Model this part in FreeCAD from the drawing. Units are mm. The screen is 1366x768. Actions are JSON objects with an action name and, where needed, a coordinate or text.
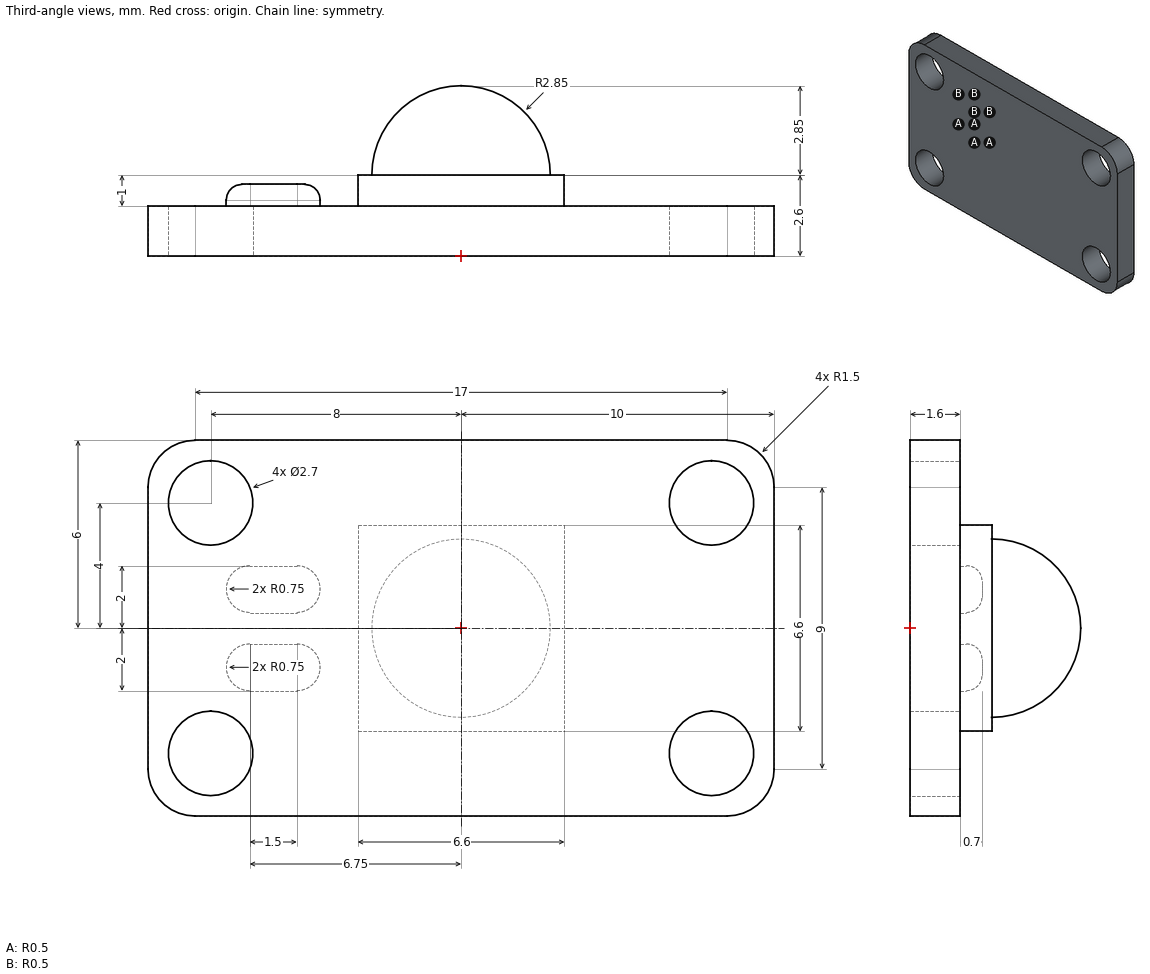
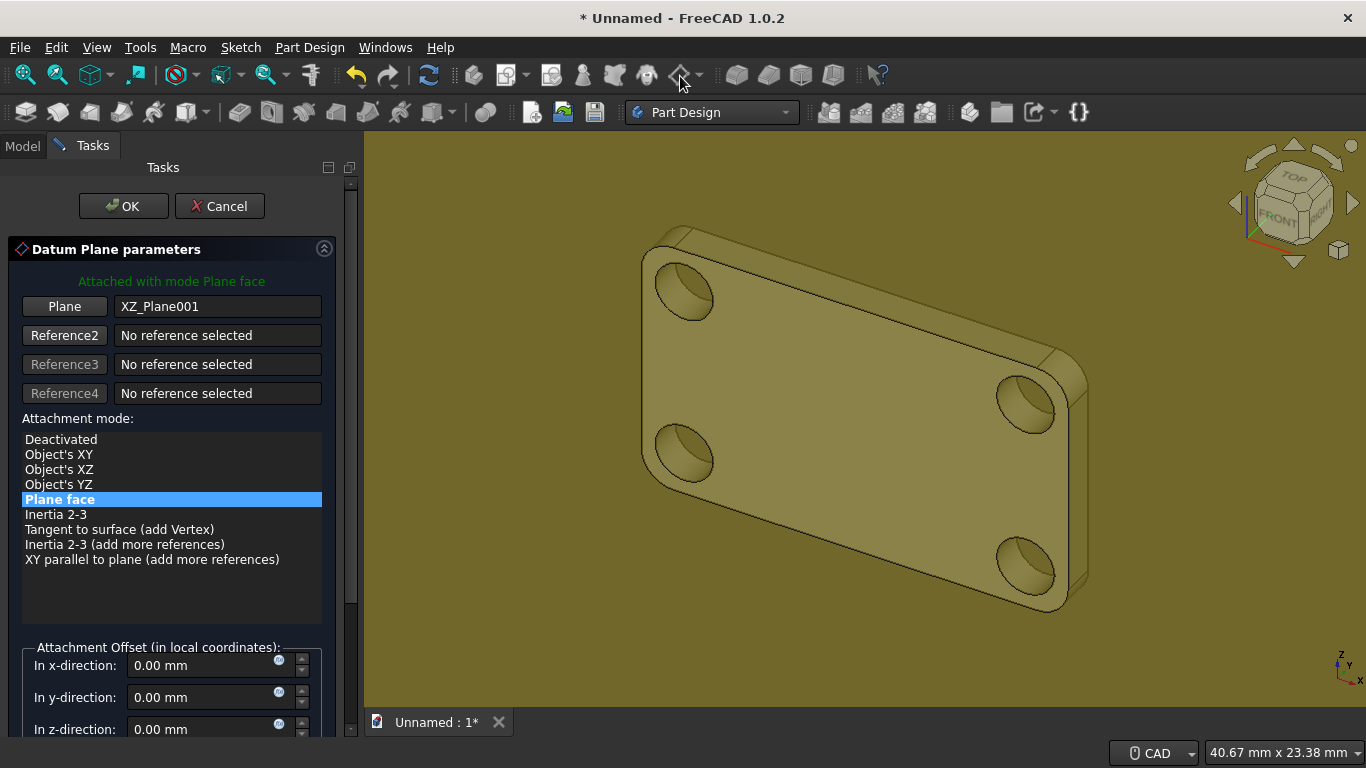
{"action": "scroll", "coordinate": [351, 456], "scroll_direction": "down", "scroll_amount": 2}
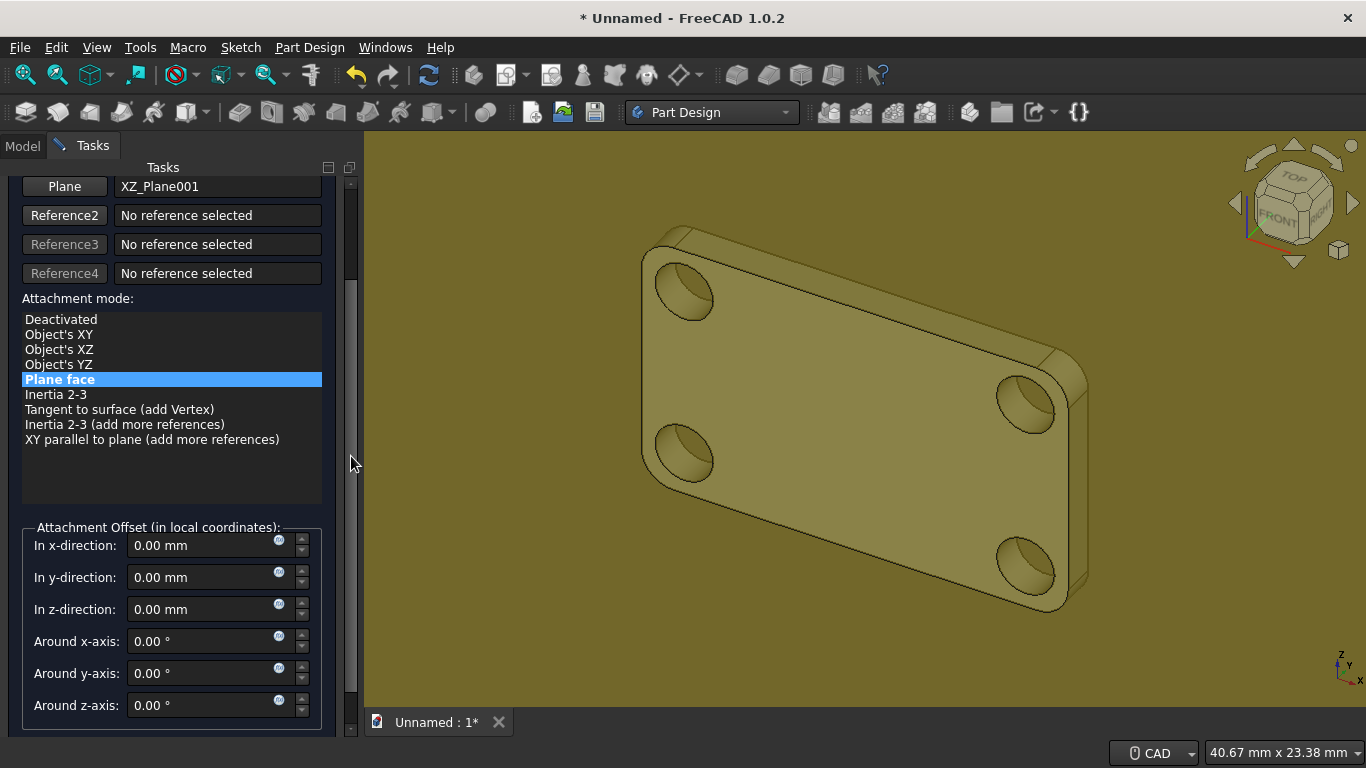
{"action": "triple_click", "coordinate": [210, 609]}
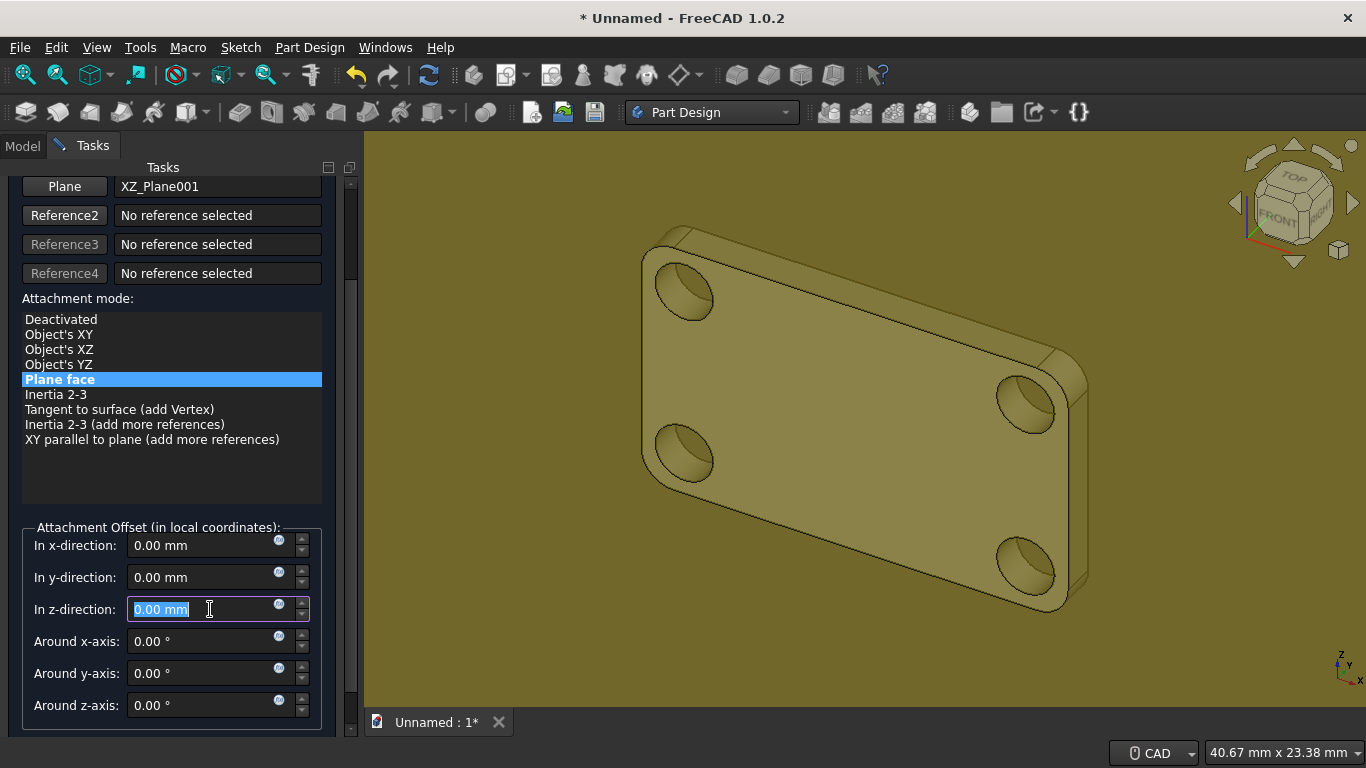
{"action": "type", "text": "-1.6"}
{"action": "key", "text": "Tab"}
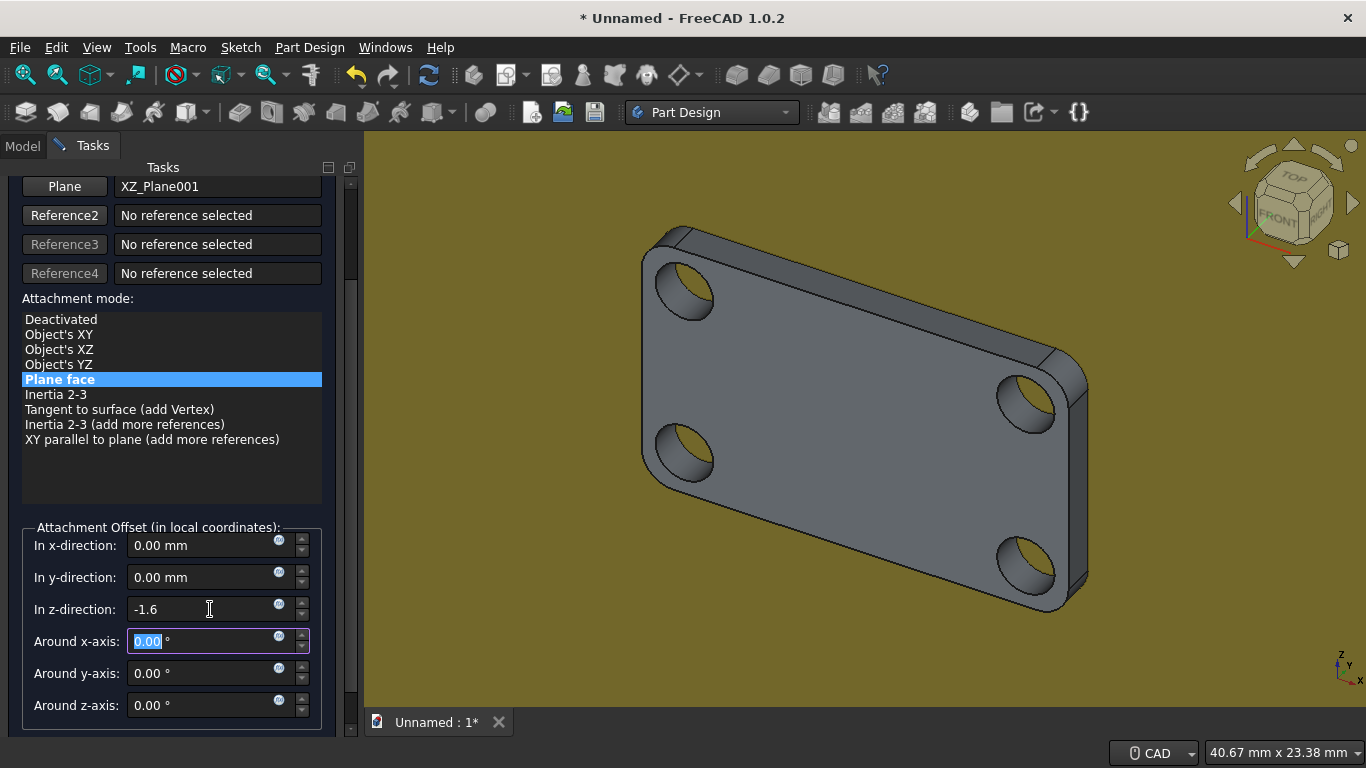
{"action": "scroll", "coordinate": [351, 456], "scroll_direction": "up", "scroll_amount": 3}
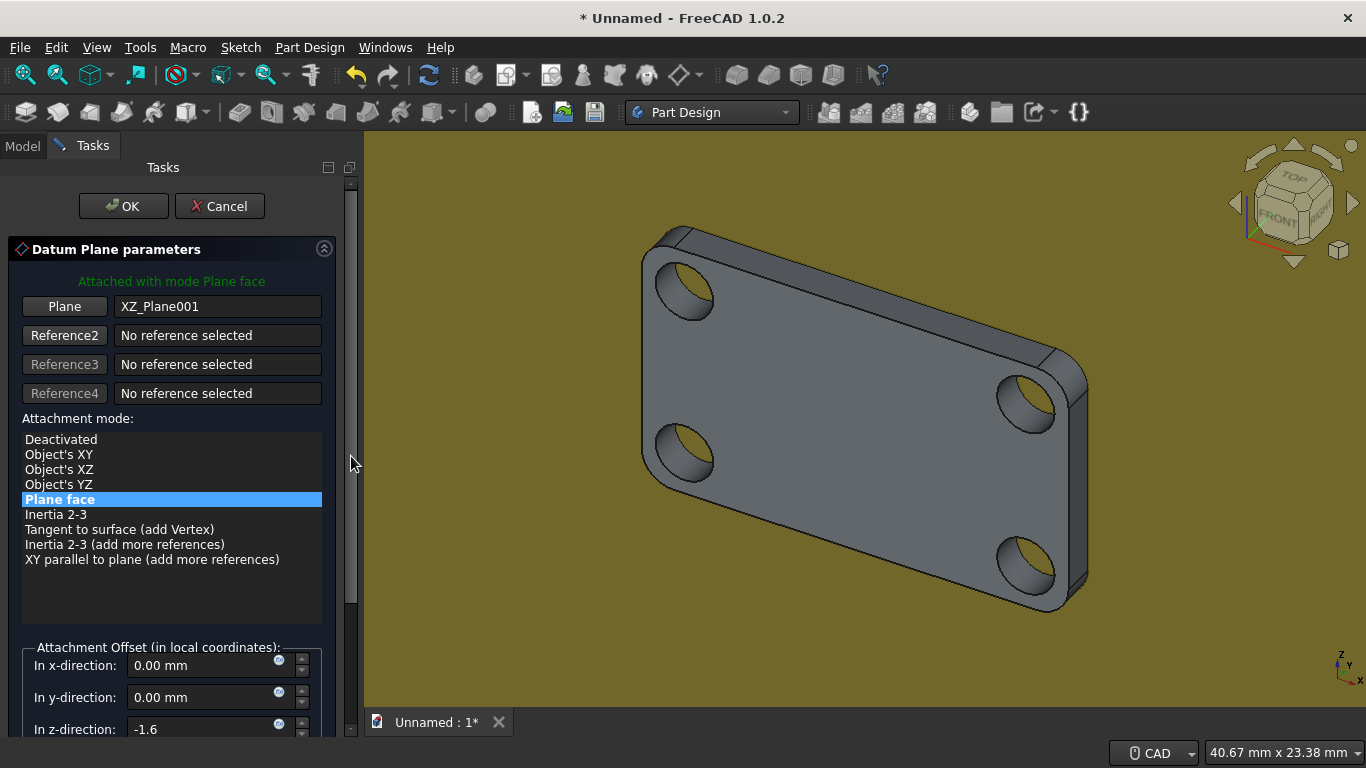
{"action": "left_click", "coordinate": [124, 206]}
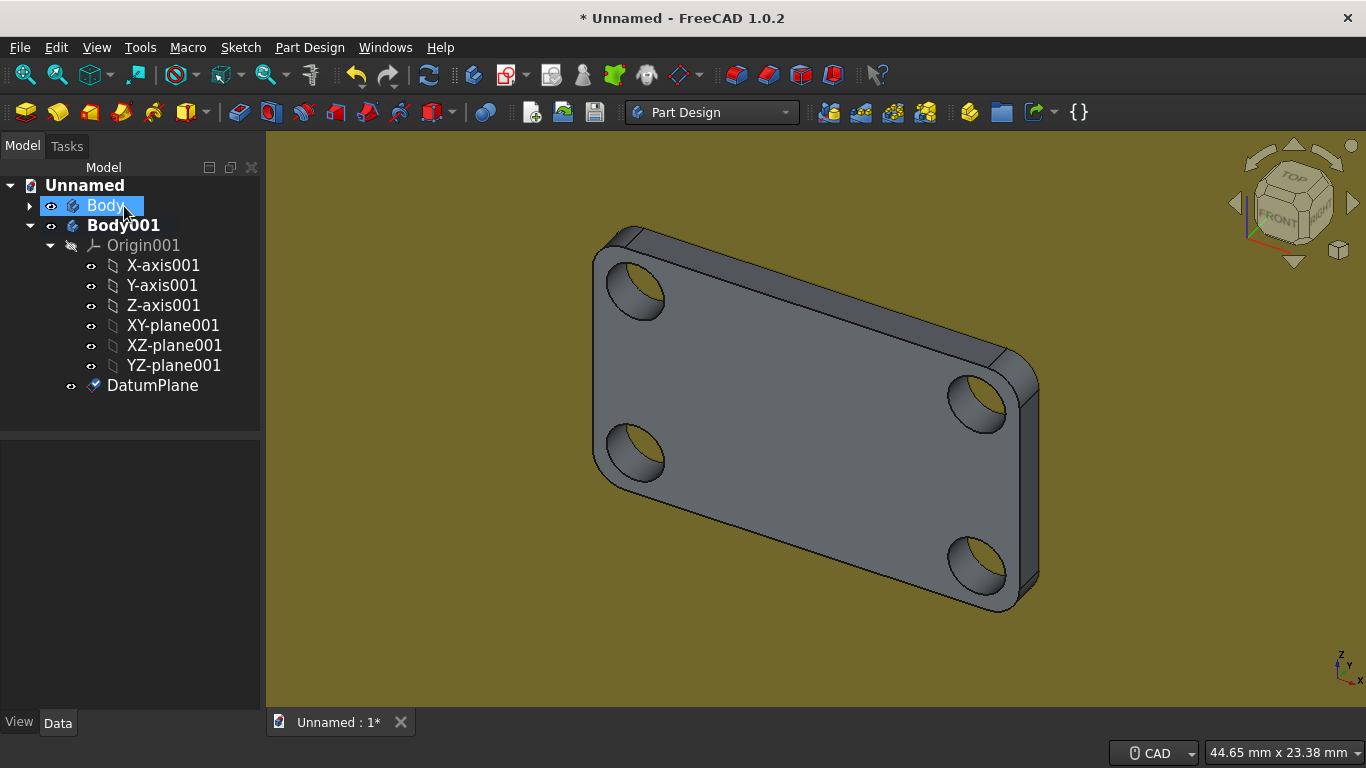
{"action": "left_click", "coordinate": [116, 386]}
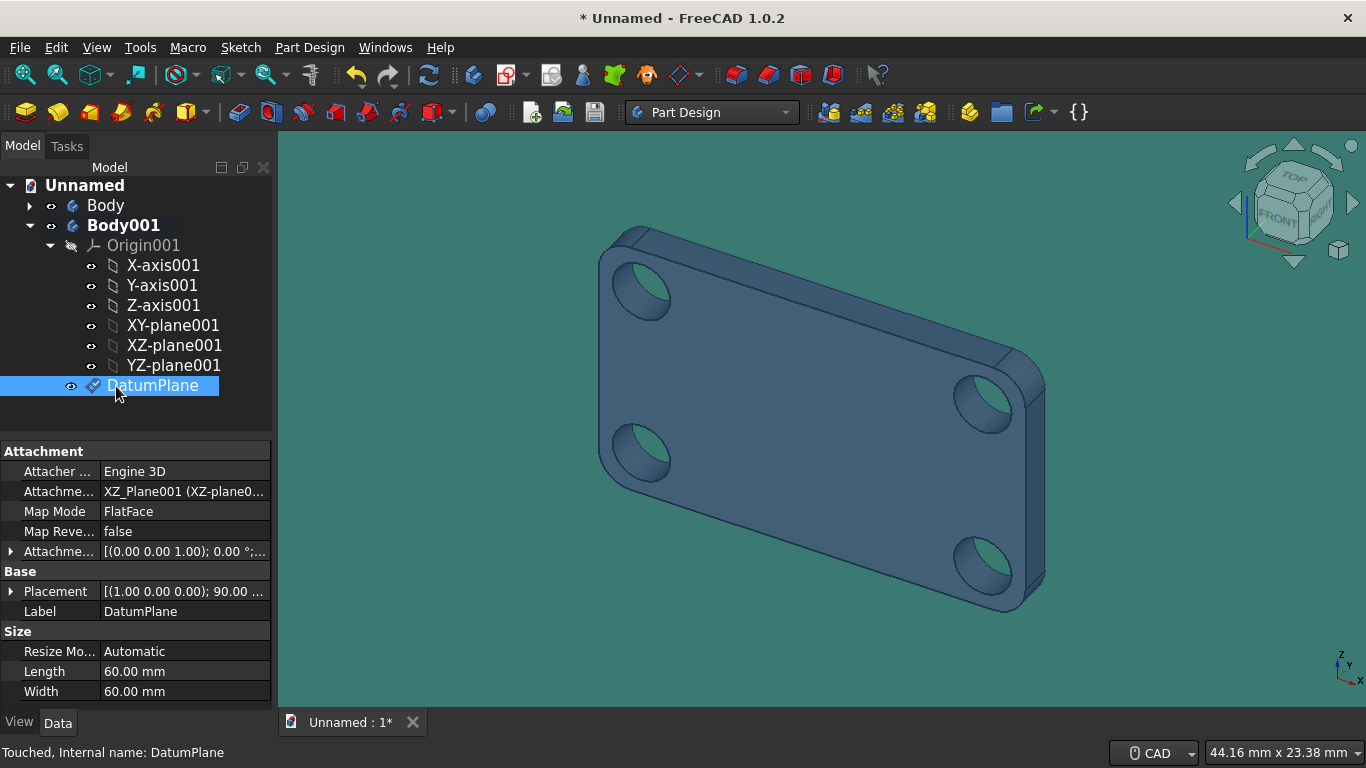
{"action": "left_click", "coordinate": [506, 76]}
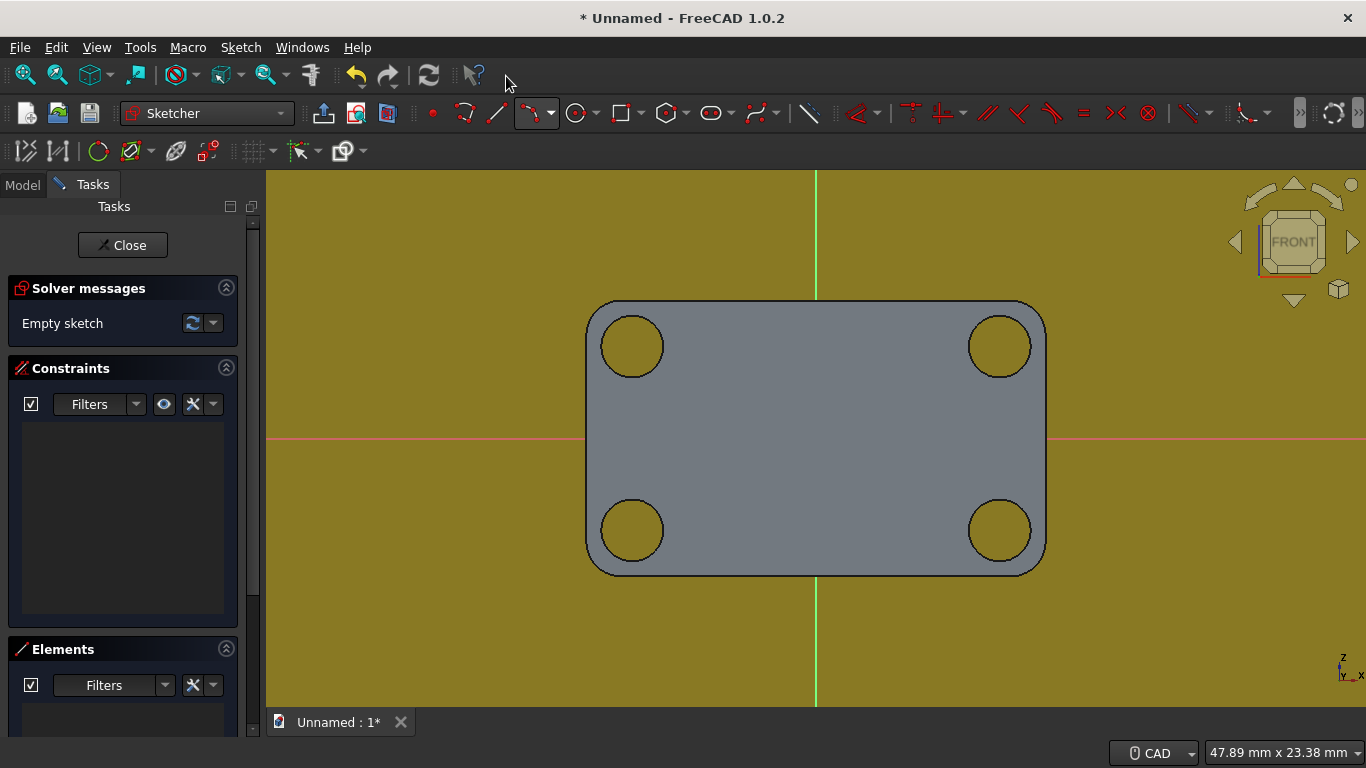
{"action": "scroll", "coordinate": [872, 438], "scroll_direction": "up", "scroll_amount": 4}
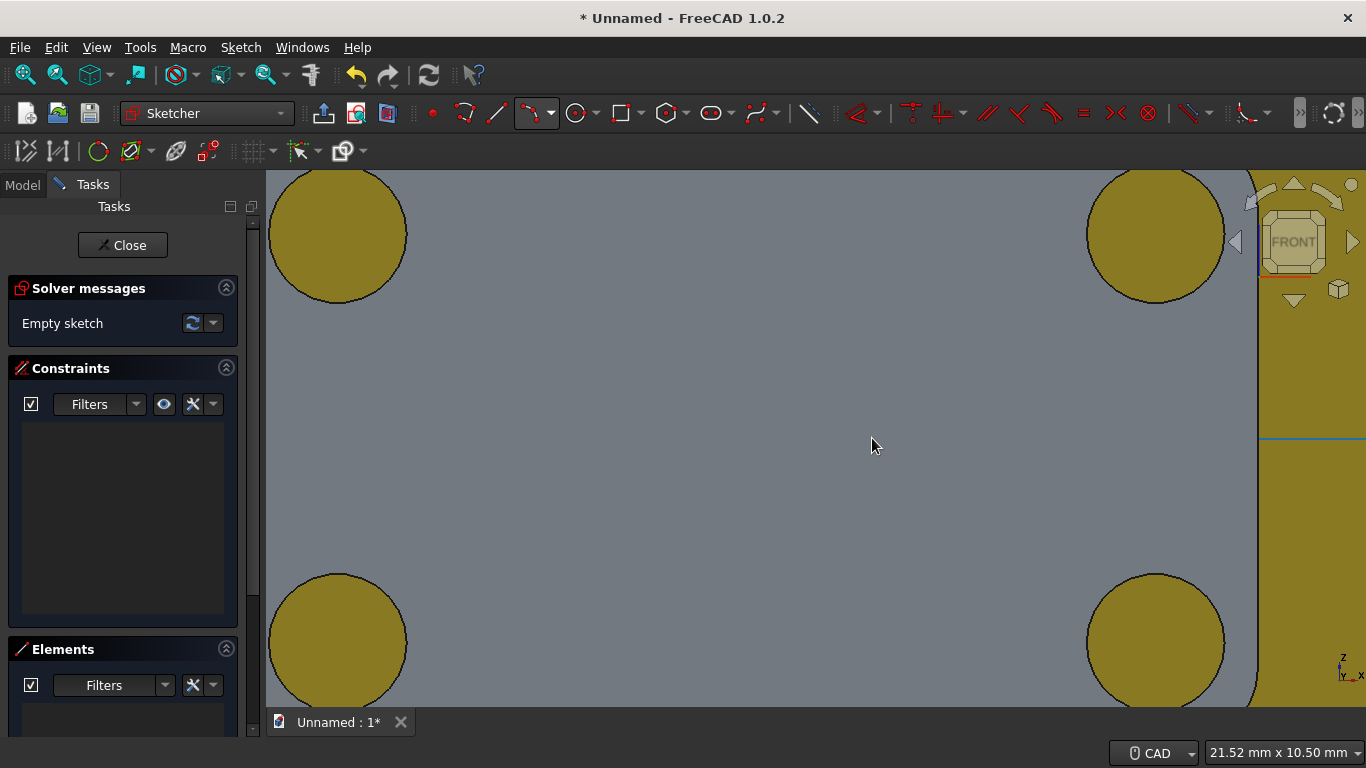
{"action": "left_click", "coordinate": [644, 114]}